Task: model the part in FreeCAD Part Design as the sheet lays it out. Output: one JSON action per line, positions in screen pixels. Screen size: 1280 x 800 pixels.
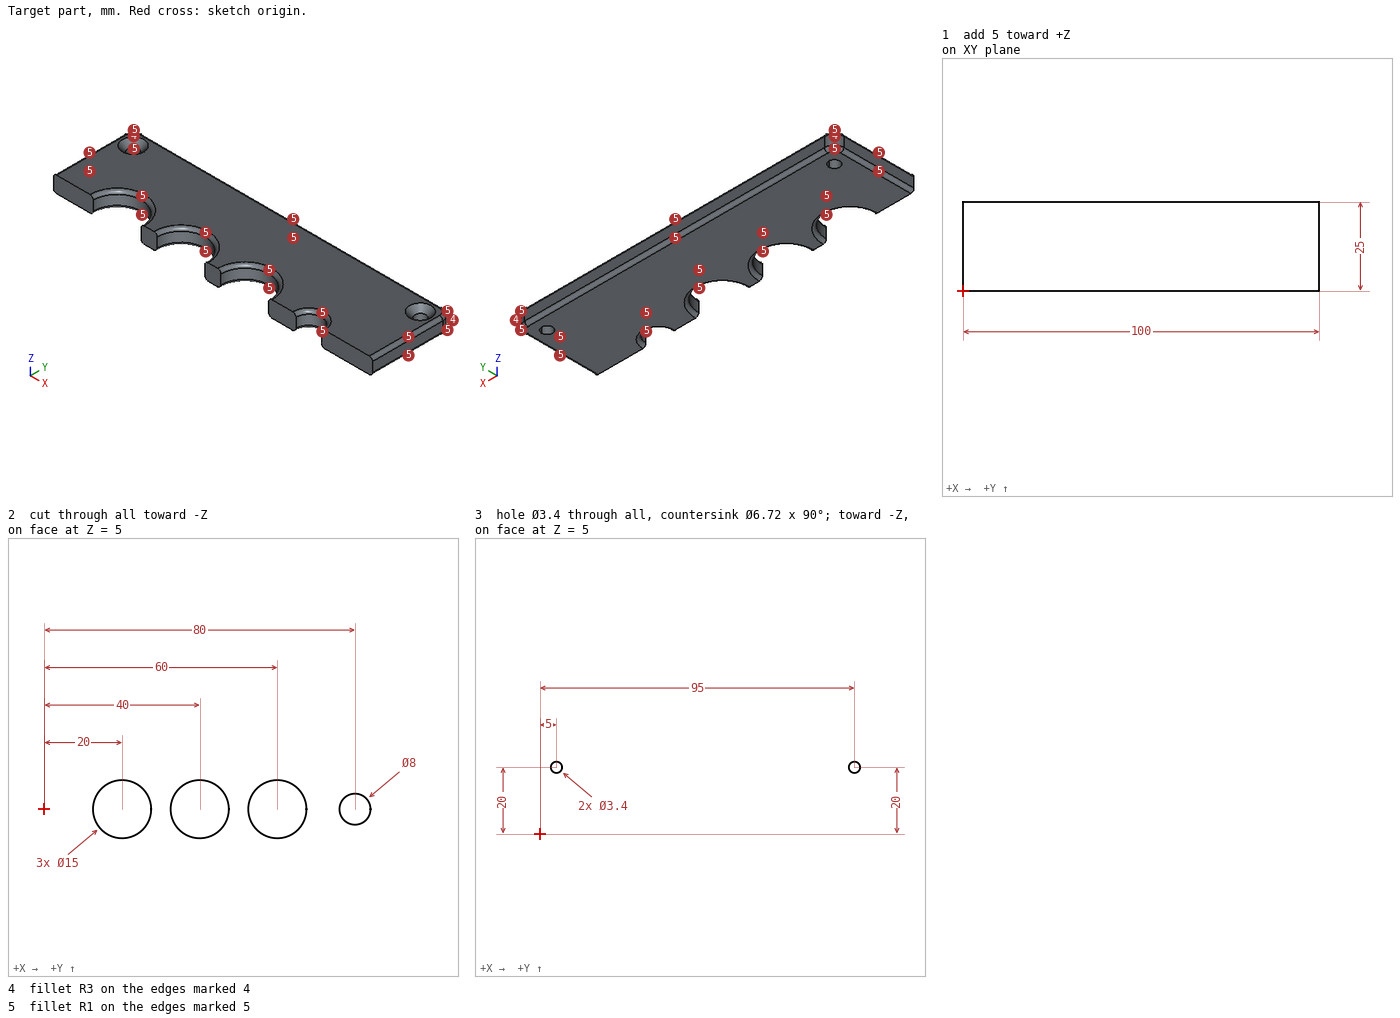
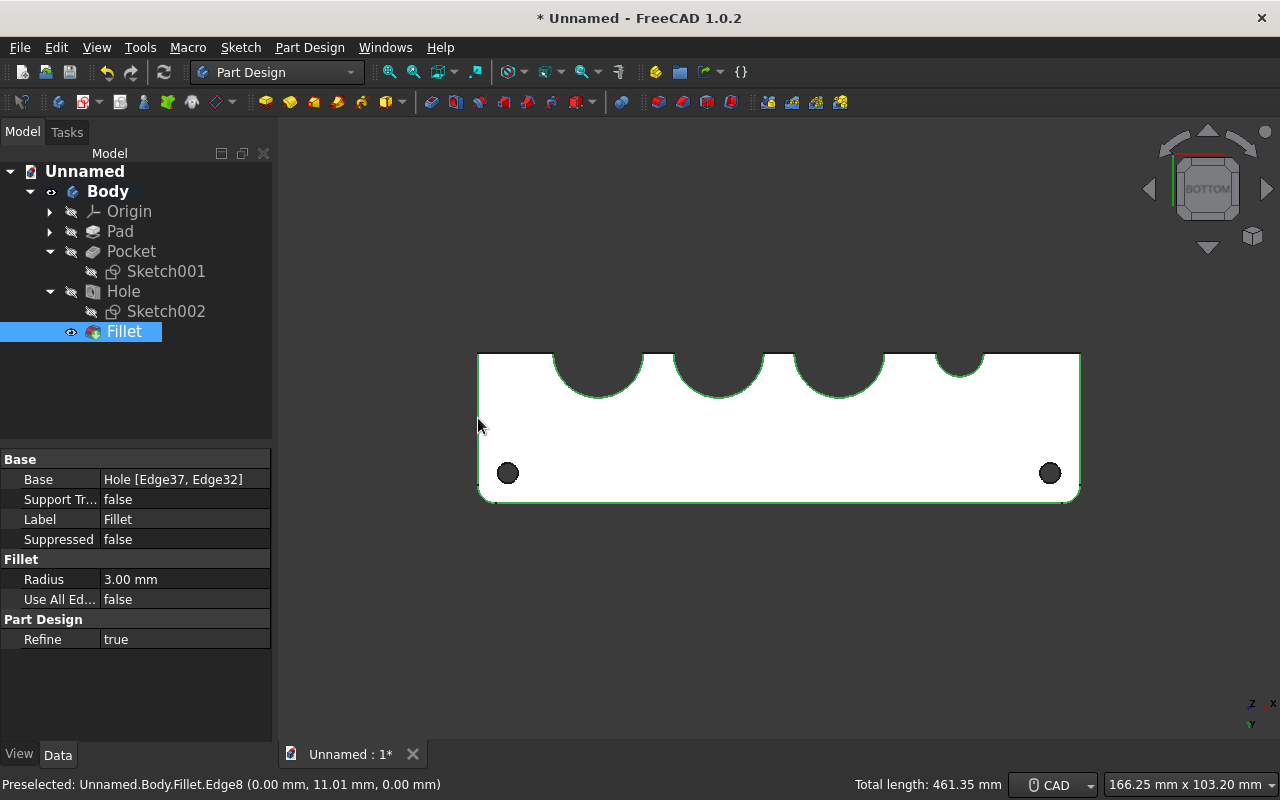
{"action": "left_click", "coordinate": [660, 102]}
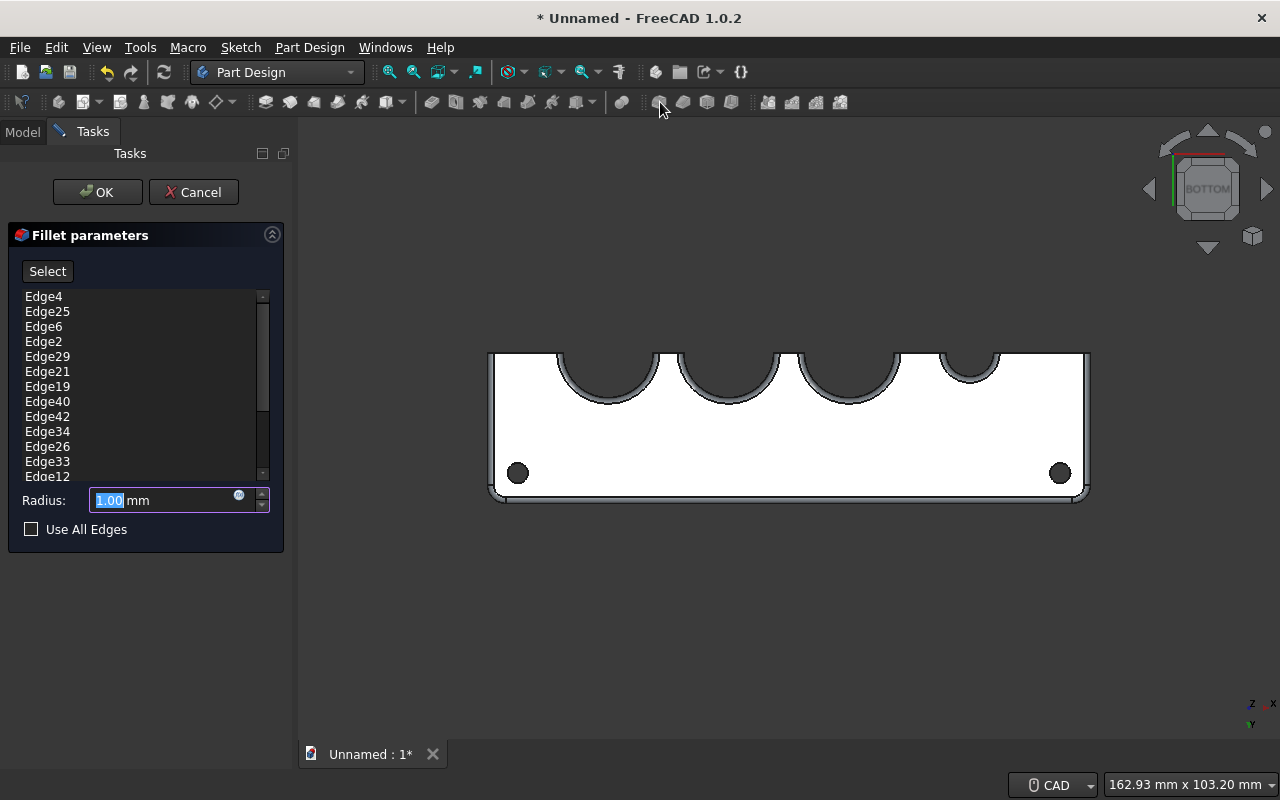
{"action": "type", "text": "1"}
{"action": "key", "text": "Tab"}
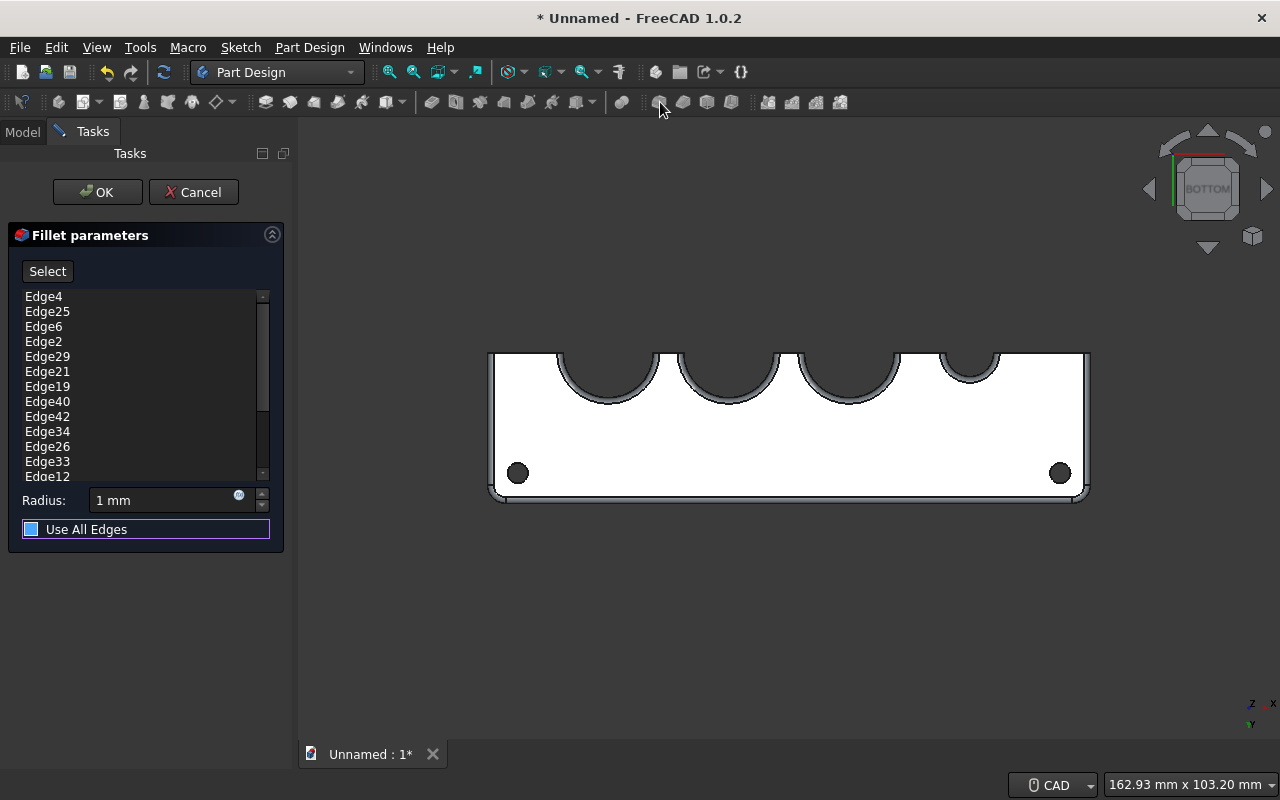
{"action": "left_click", "coordinate": [98, 192]}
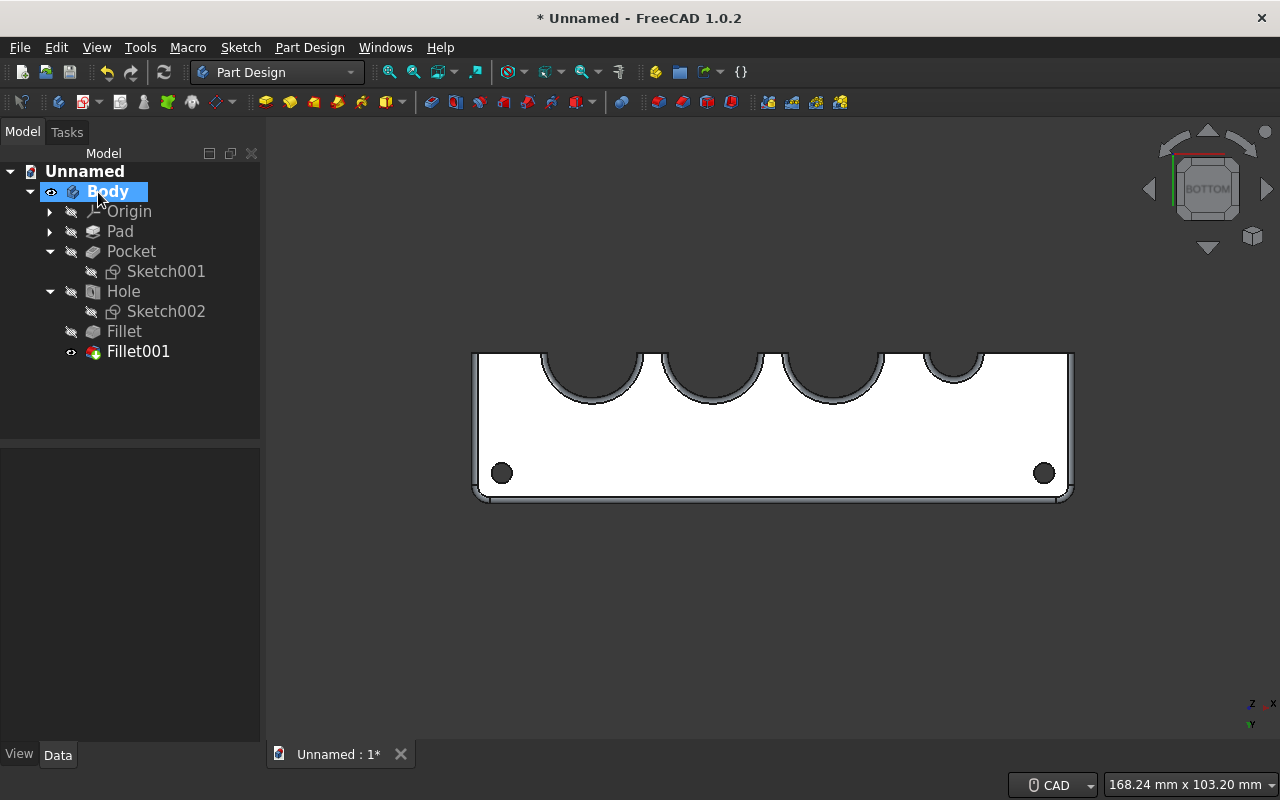
{"action": "key", "text": "0"}